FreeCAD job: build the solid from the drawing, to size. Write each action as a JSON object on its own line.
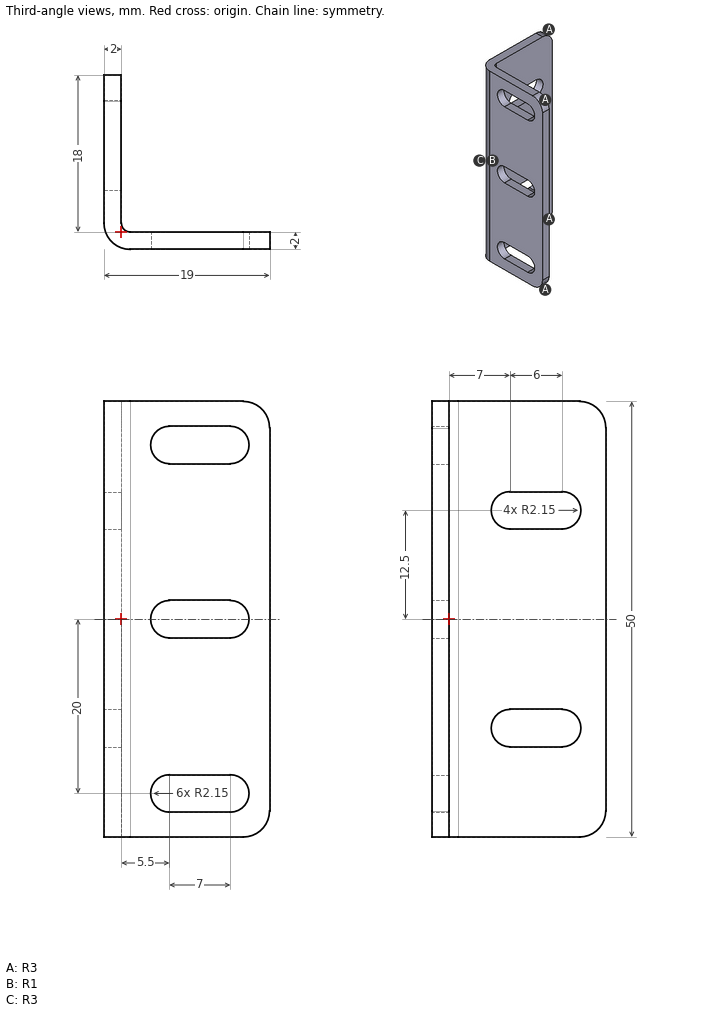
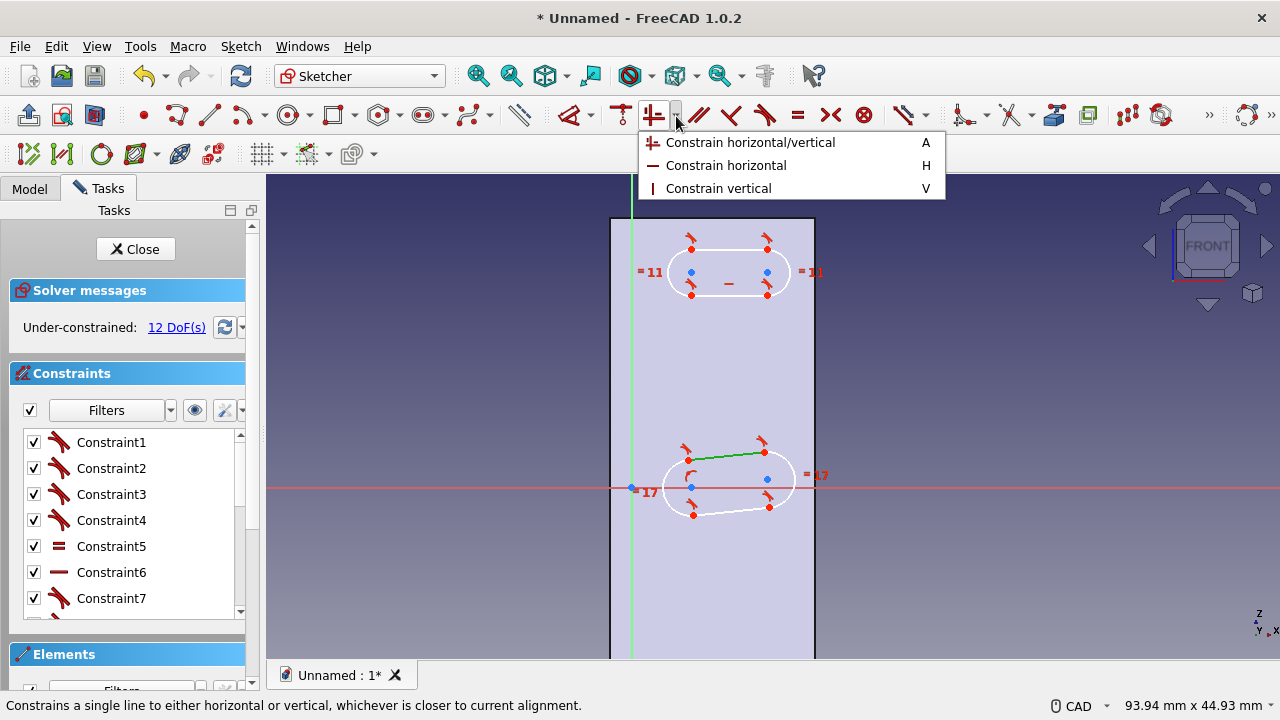
{"action": "left_click", "coordinate": [792, 166]}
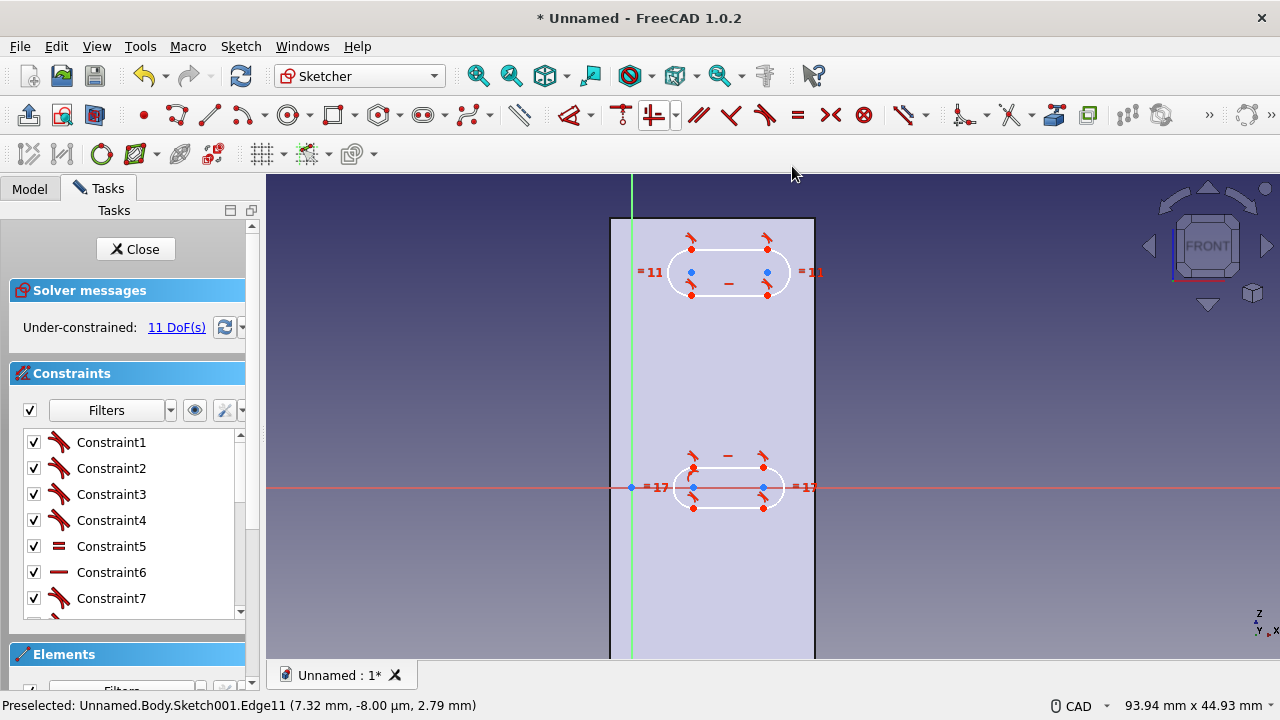
{"action": "scroll", "coordinate": [691, 271], "scroll_direction": "down", "scroll_amount": 2}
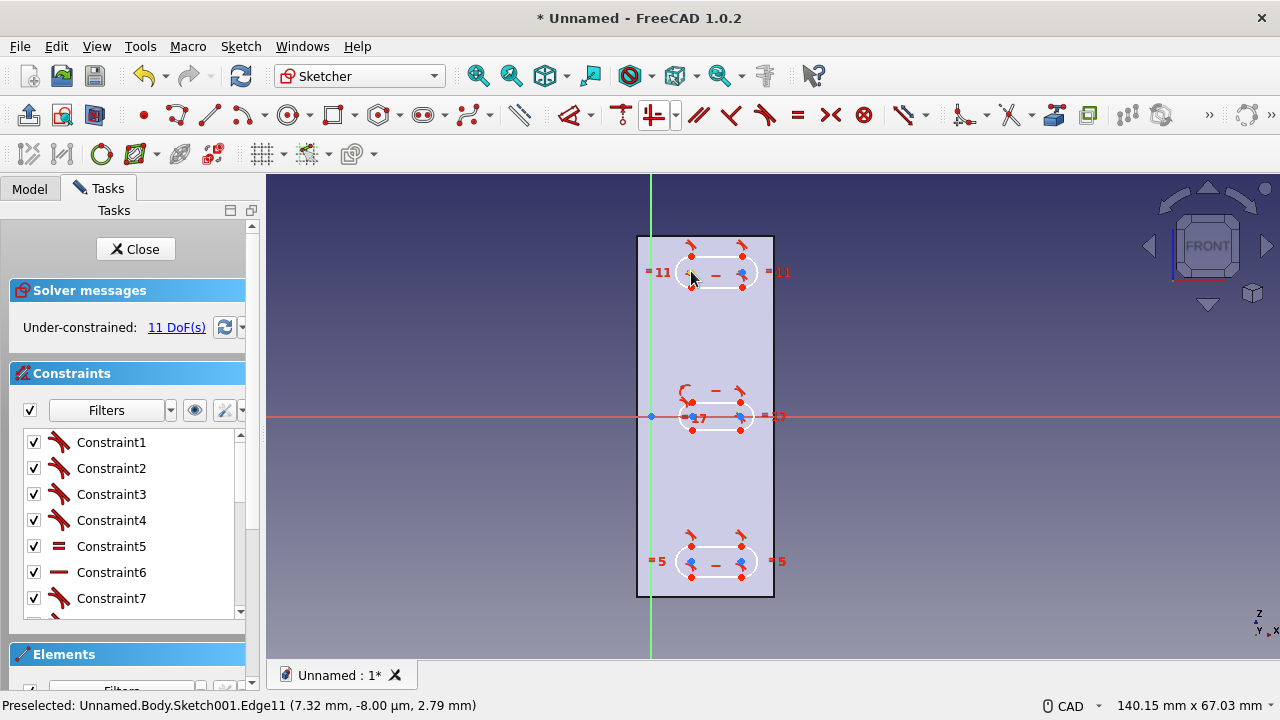
{"action": "left_click", "coordinate": [679, 553]}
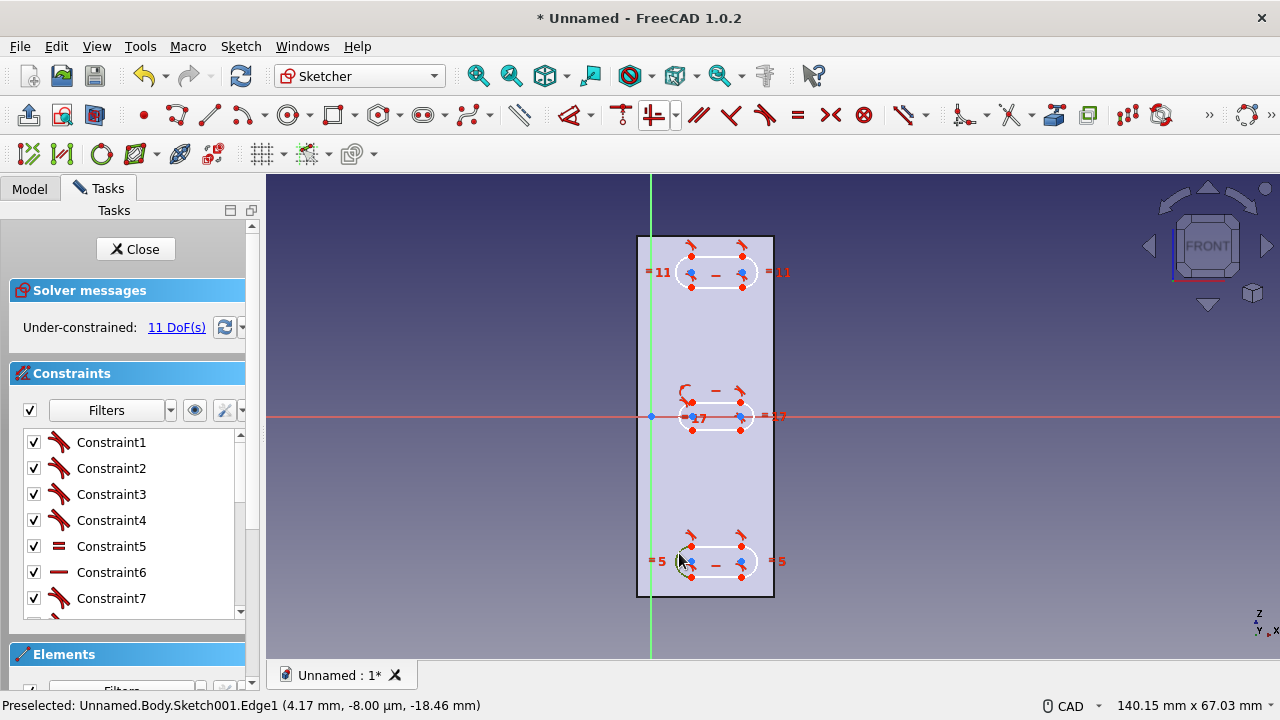
{"action": "left_click", "coordinate": [679, 263]}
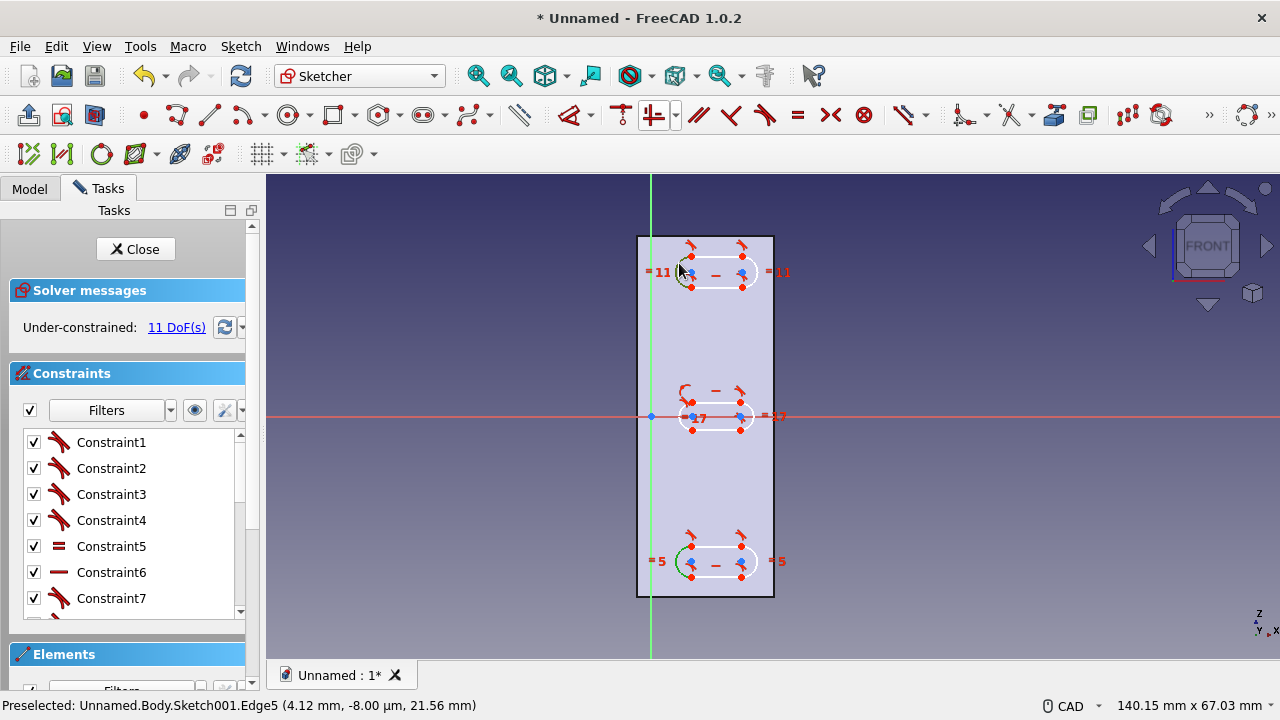
{"action": "left_click", "coordinate": [679, 416]}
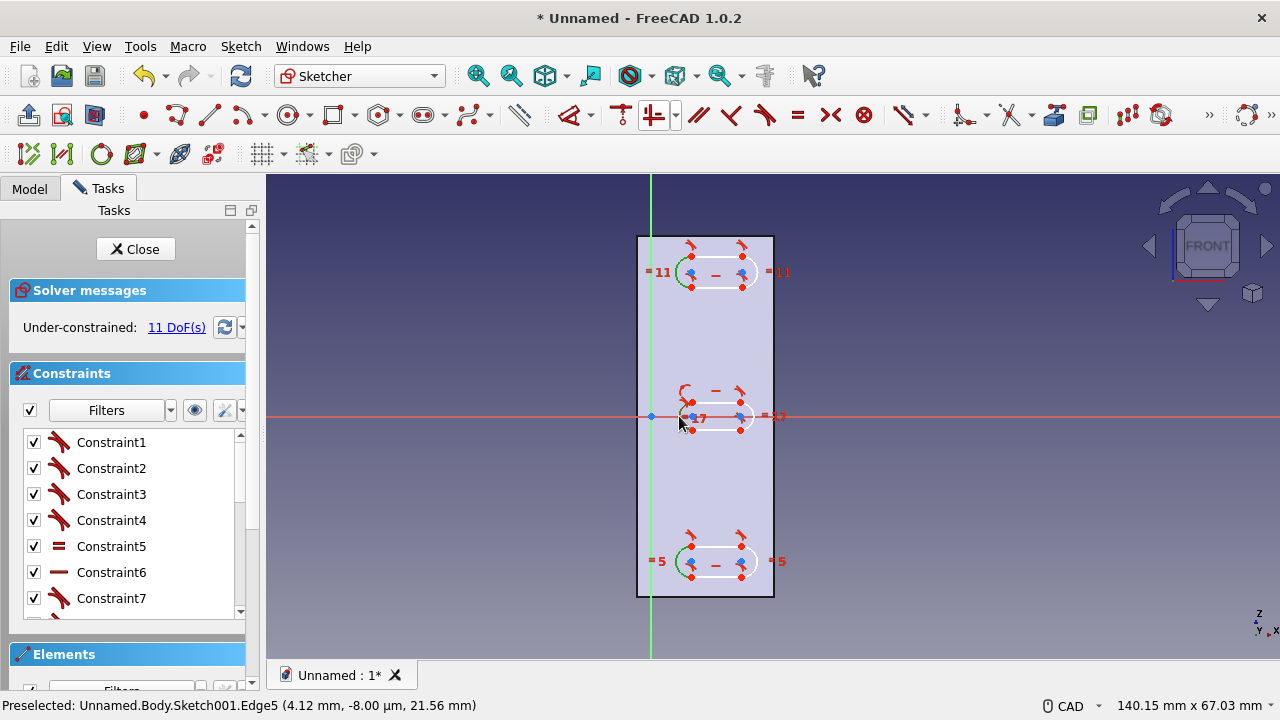
{"action": "left_click", "coordinate": [798, 116]}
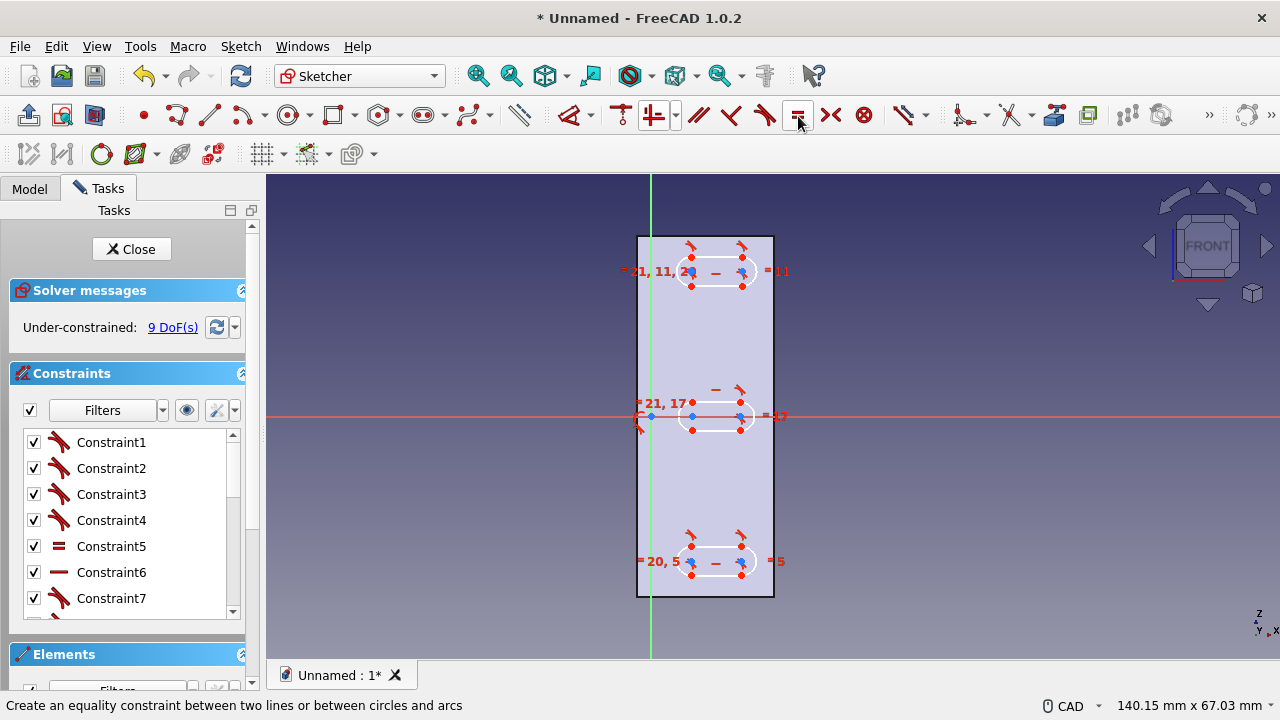
{"action": "left_click", "coordinate": [691, 561]}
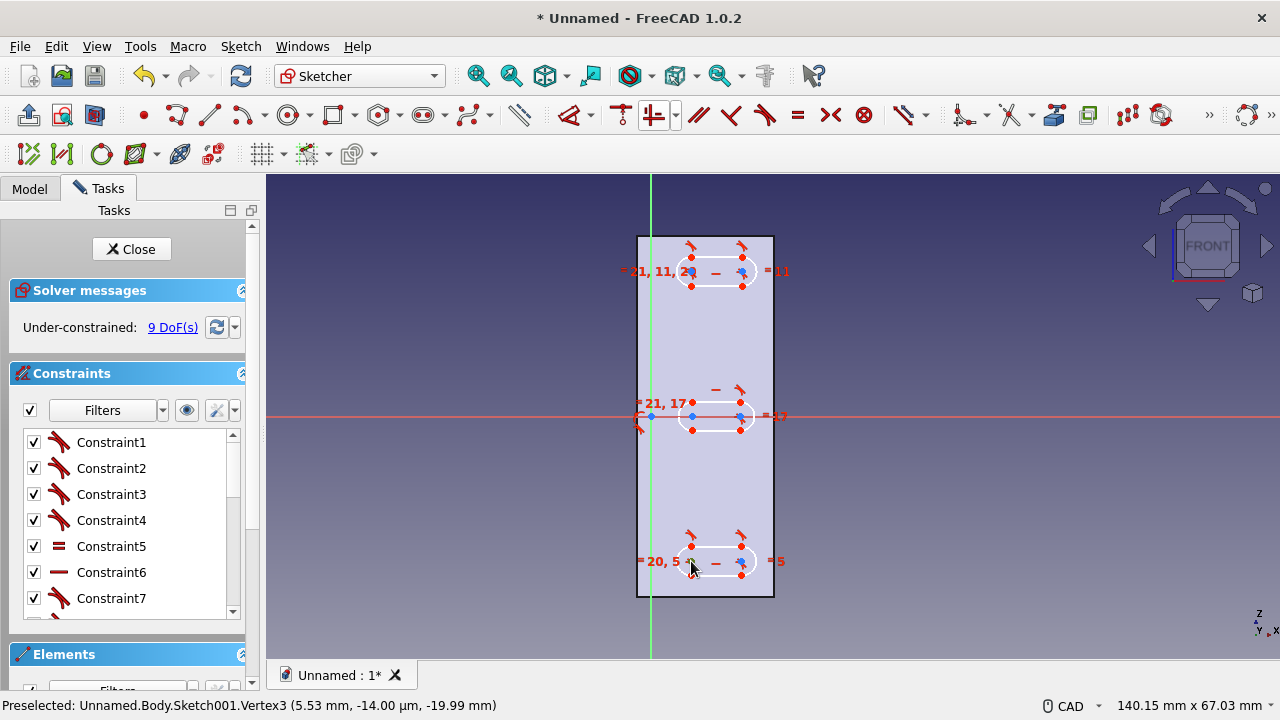
{"action": "left_click", "coordinate": [691, 272]}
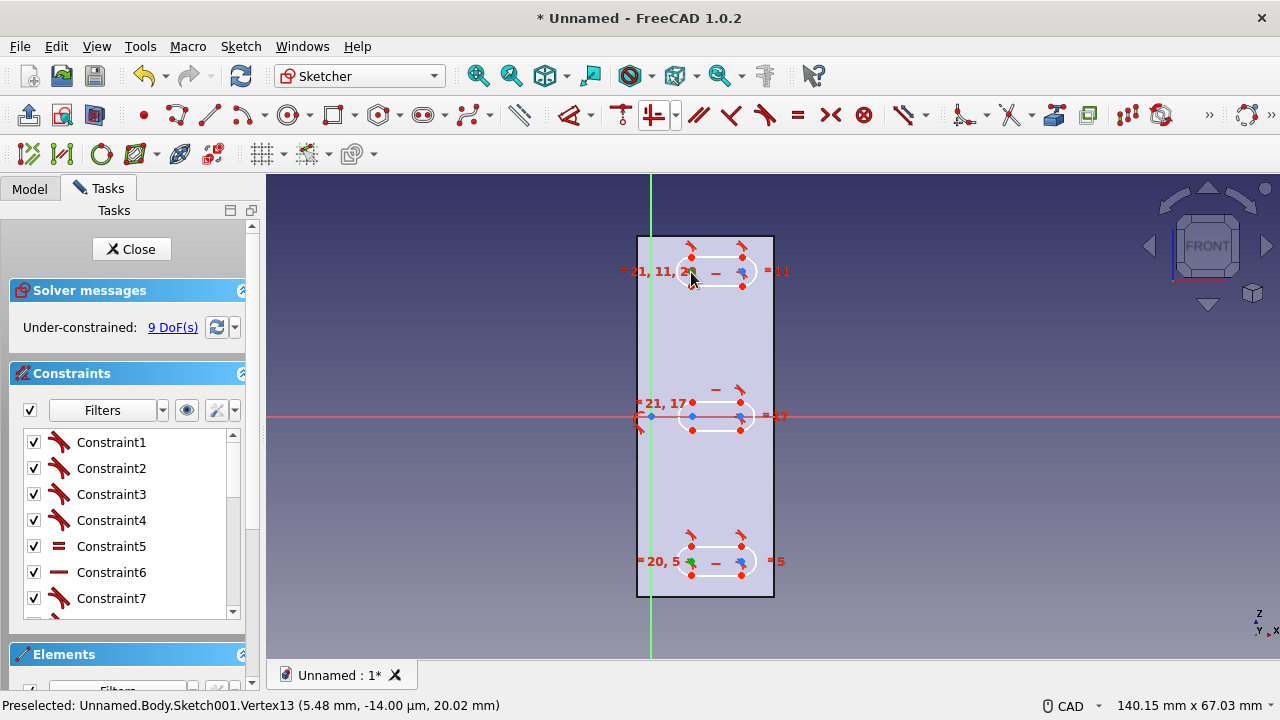
{"action": "left_click", "coordinate": [353, 416]}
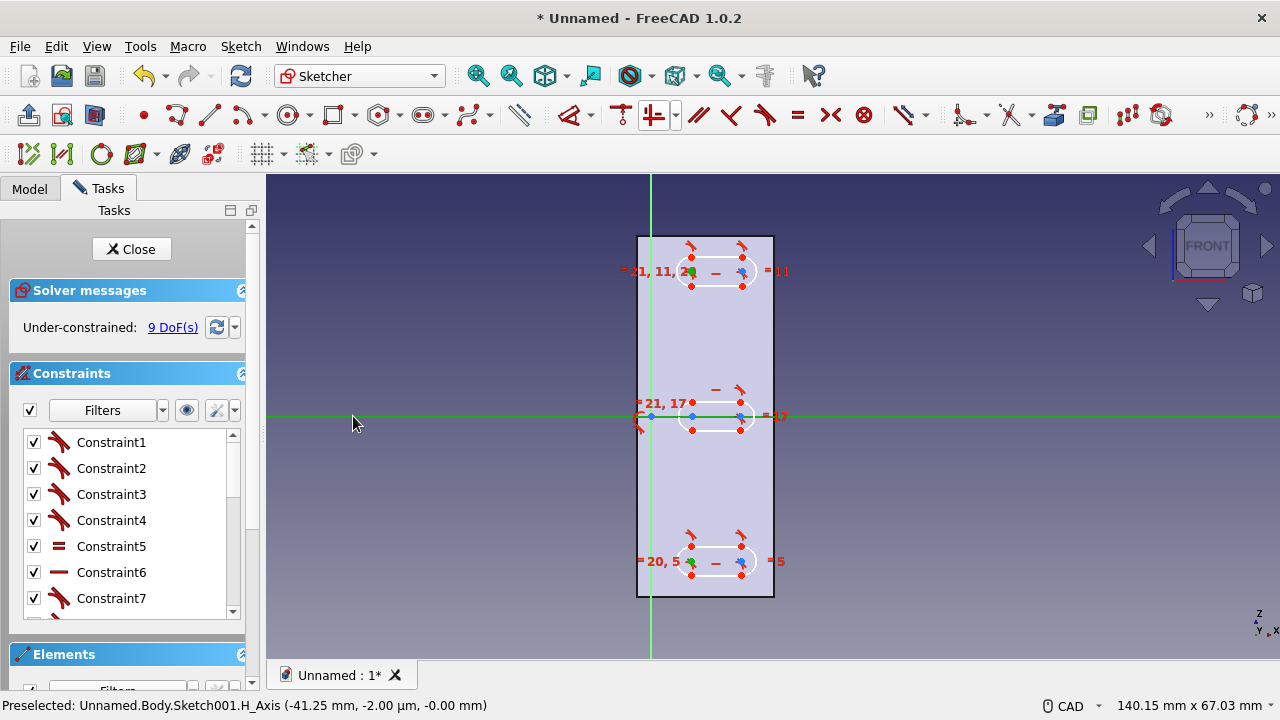
{"action": "left_click", "coordinate": [831, 116]}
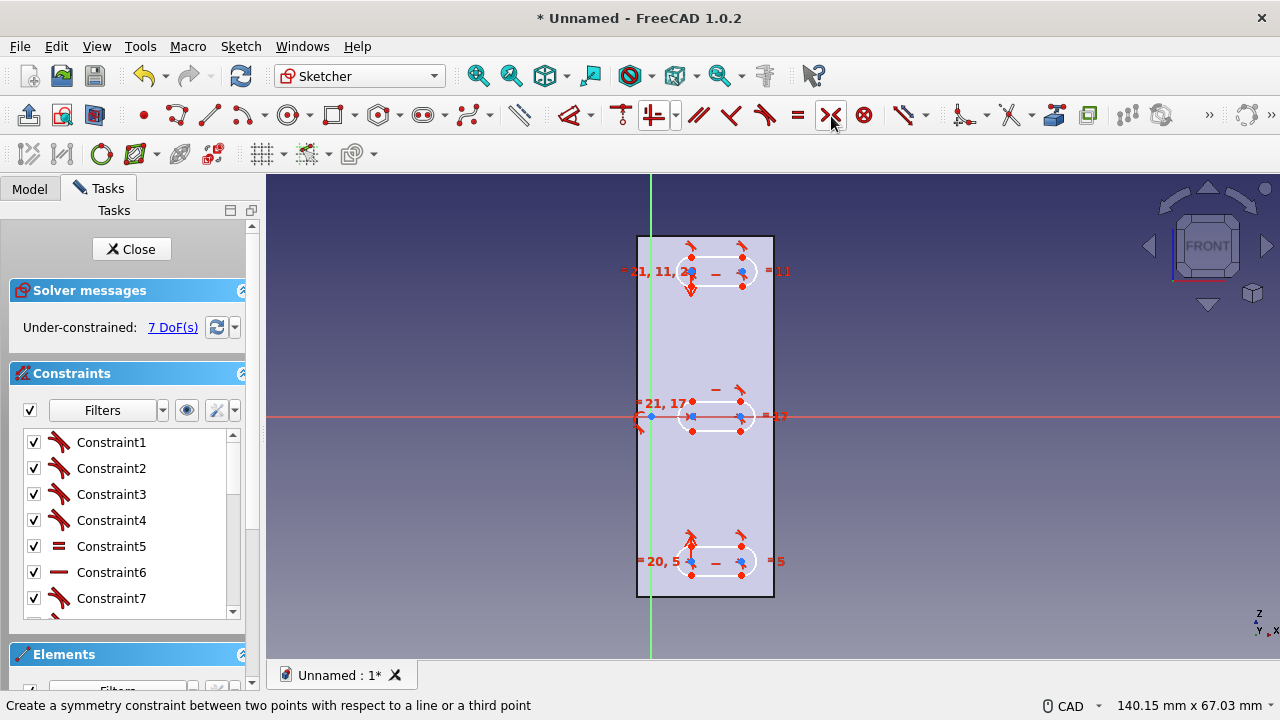
{"action": "left_click", "coordinate": [568, 116]}